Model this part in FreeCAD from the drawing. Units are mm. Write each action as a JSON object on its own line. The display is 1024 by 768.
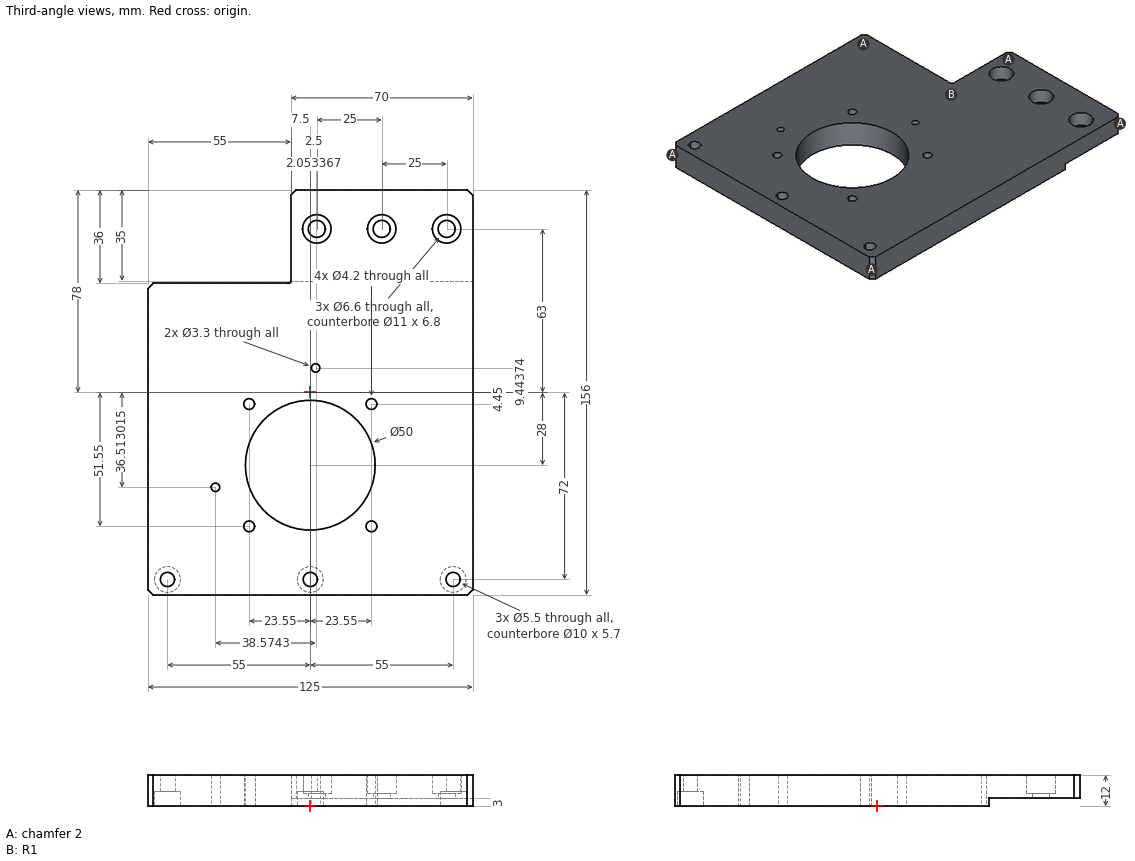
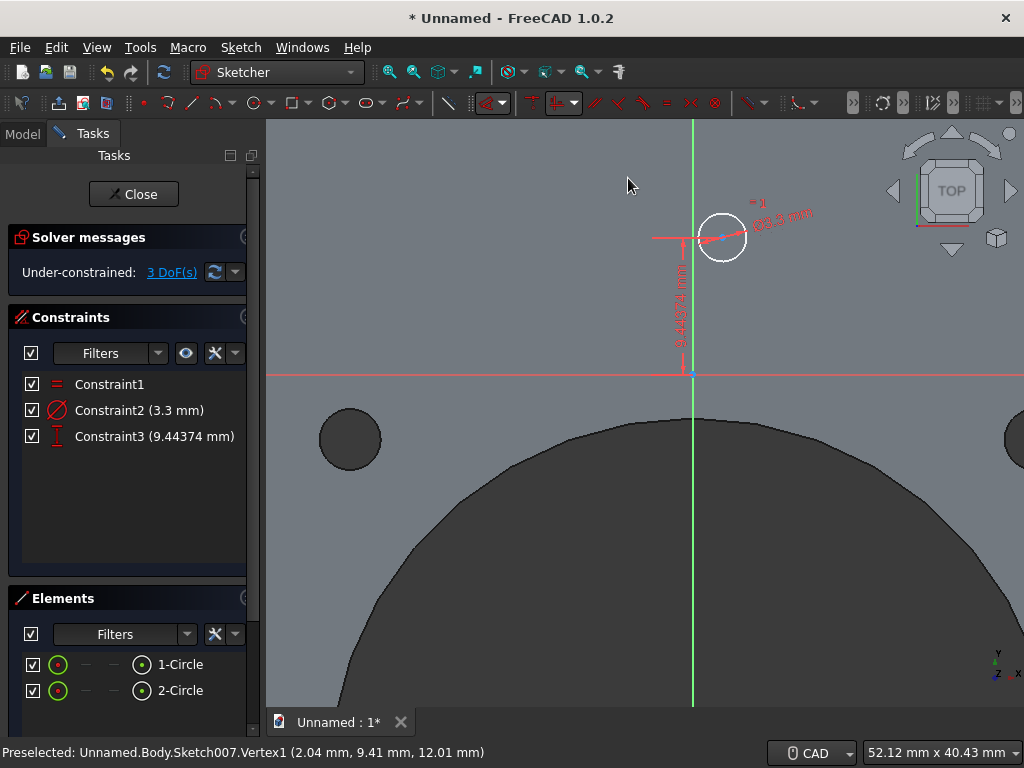
{"action": "scroll", "coordinate": [722, 238], "scroll_direction": "up", "scroll_amount": 2}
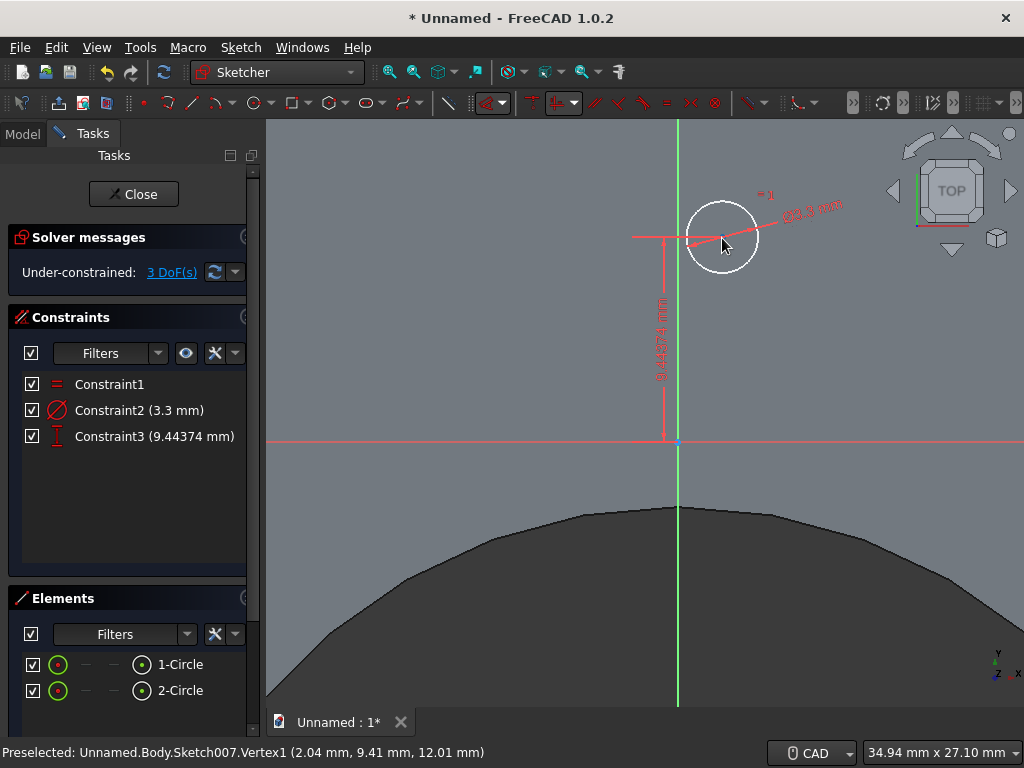
{"action": "left_click", "coordinate": [722, 237]}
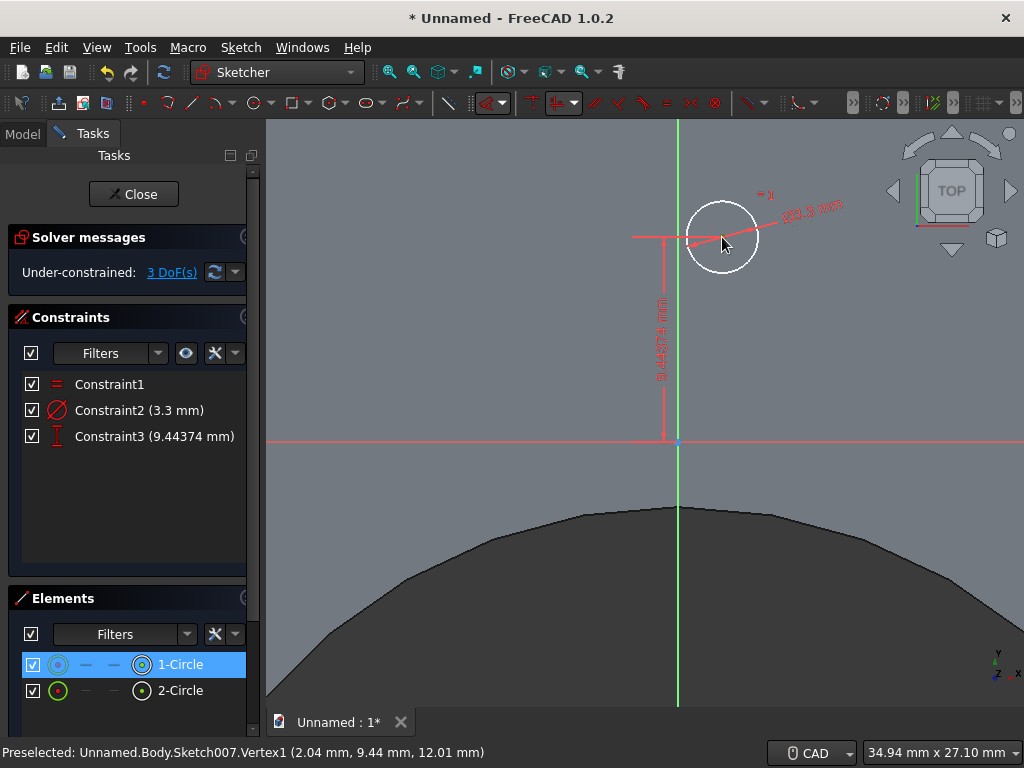
{"action": "left_click", "coordinate": [504, 104]}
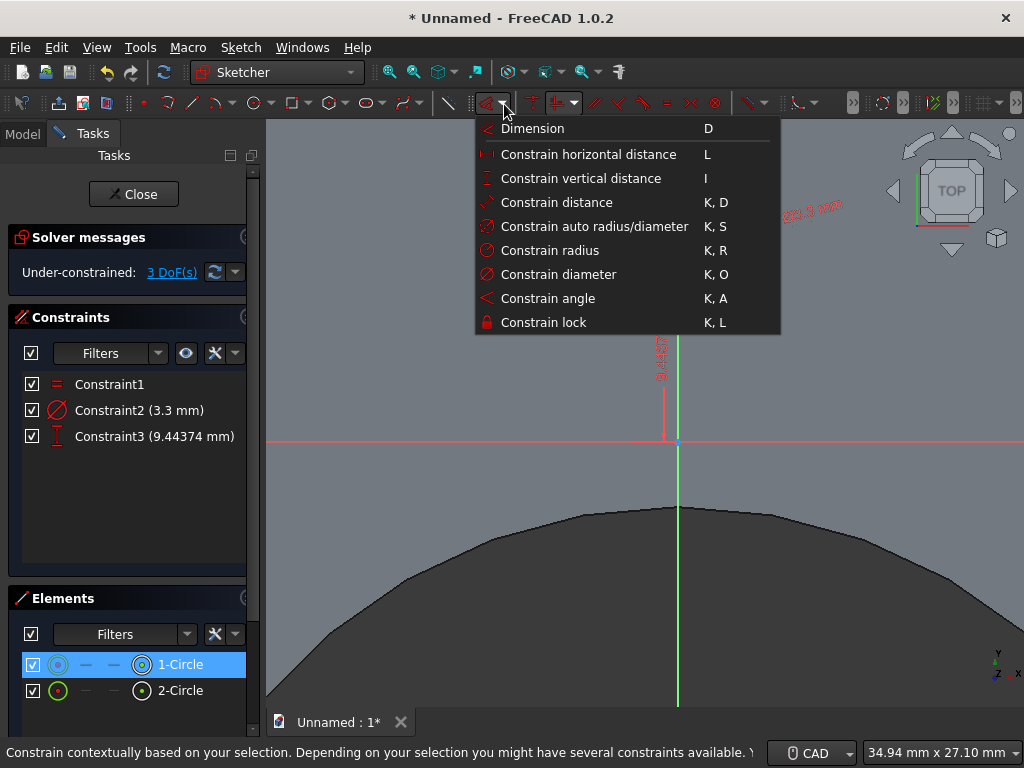
{"action": "left_click", "coordinate": [628, 154]}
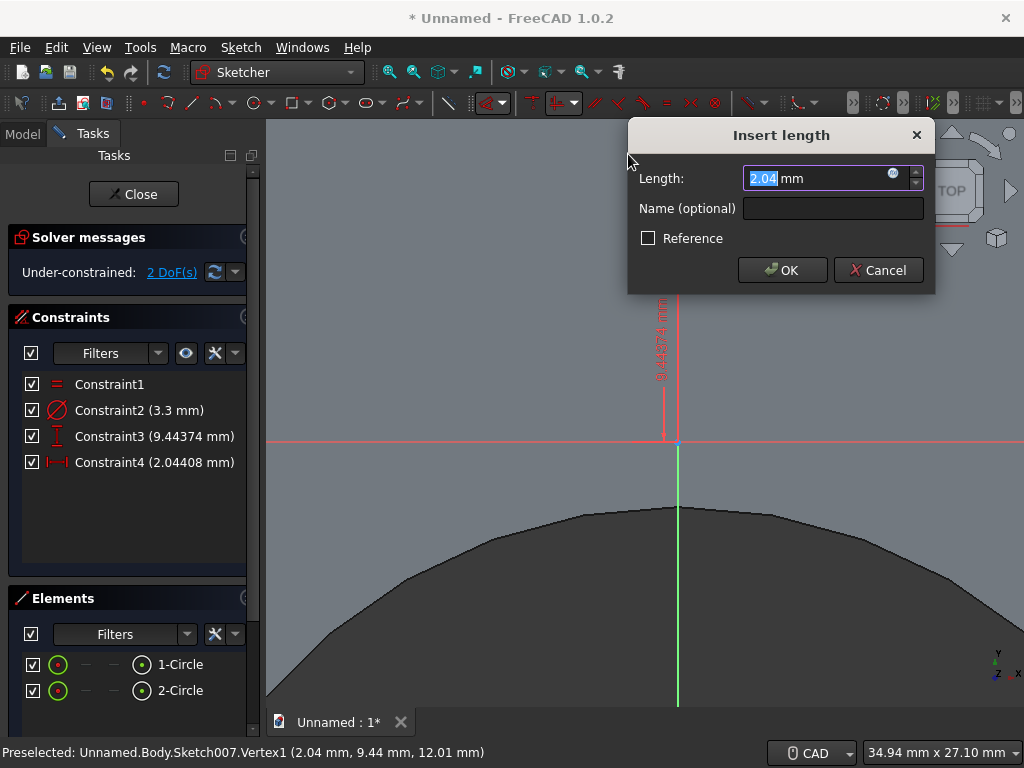
{"action": "type", "text": "2.053367"}
{"action": "key", "text": "Return"}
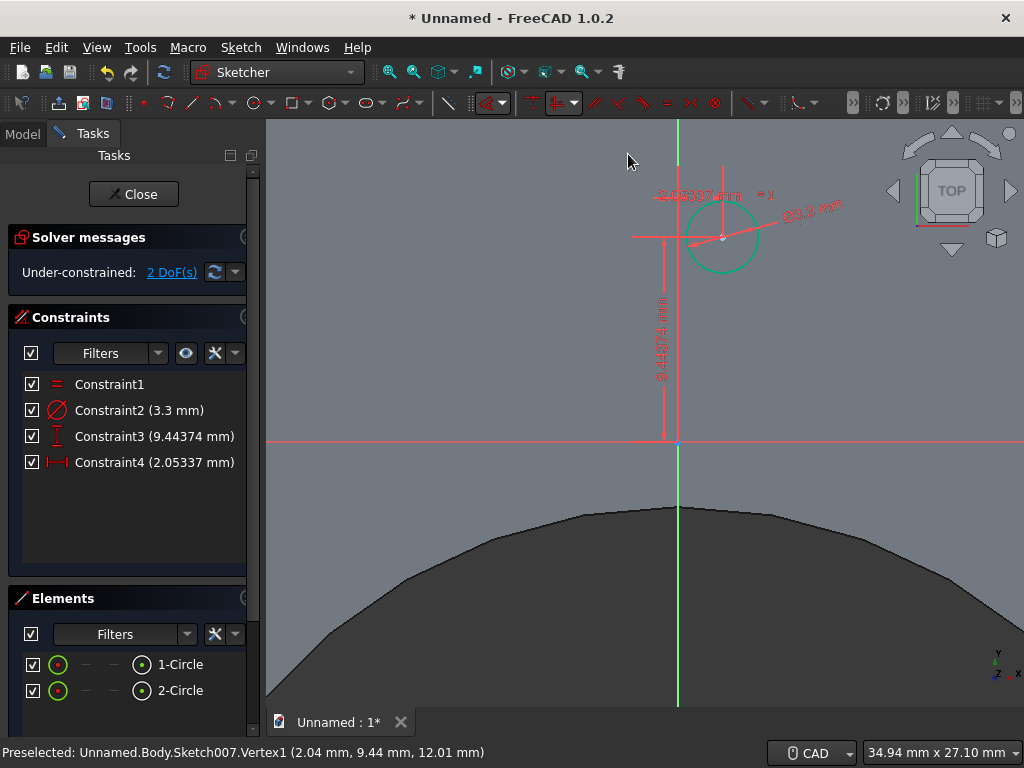
{"action": "left_click", "coordinate": [723, 237]}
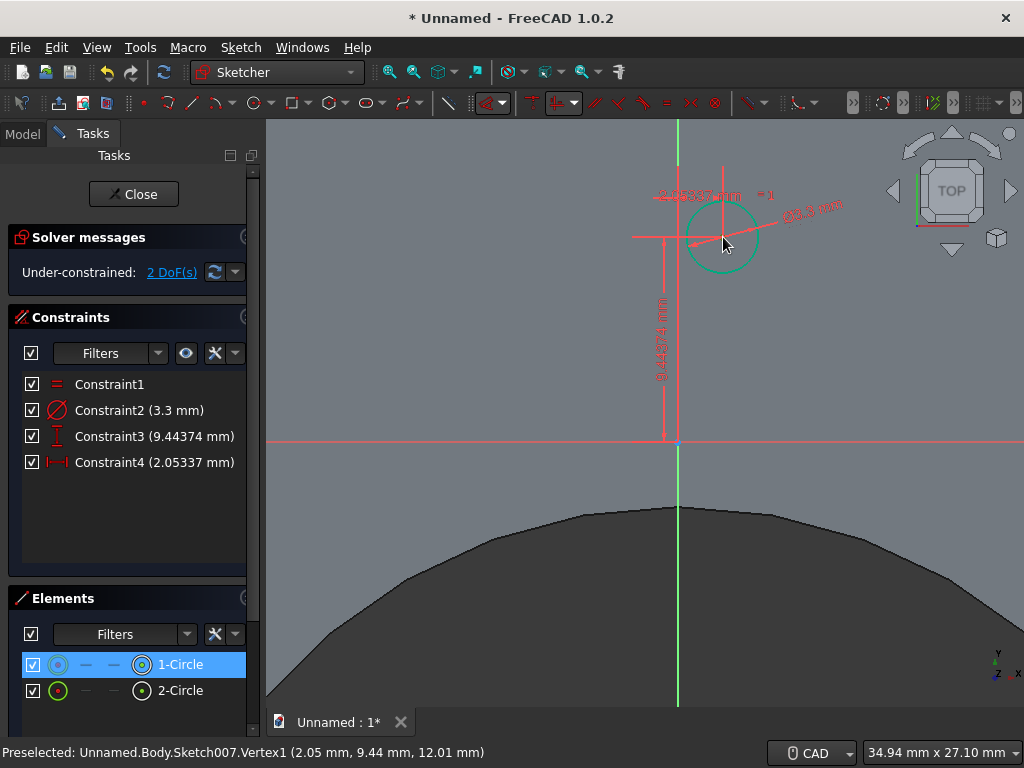
{"action": "scroll", "coordinate": [735, 225], "scroll_direction": "down", "scroll_amount": 5}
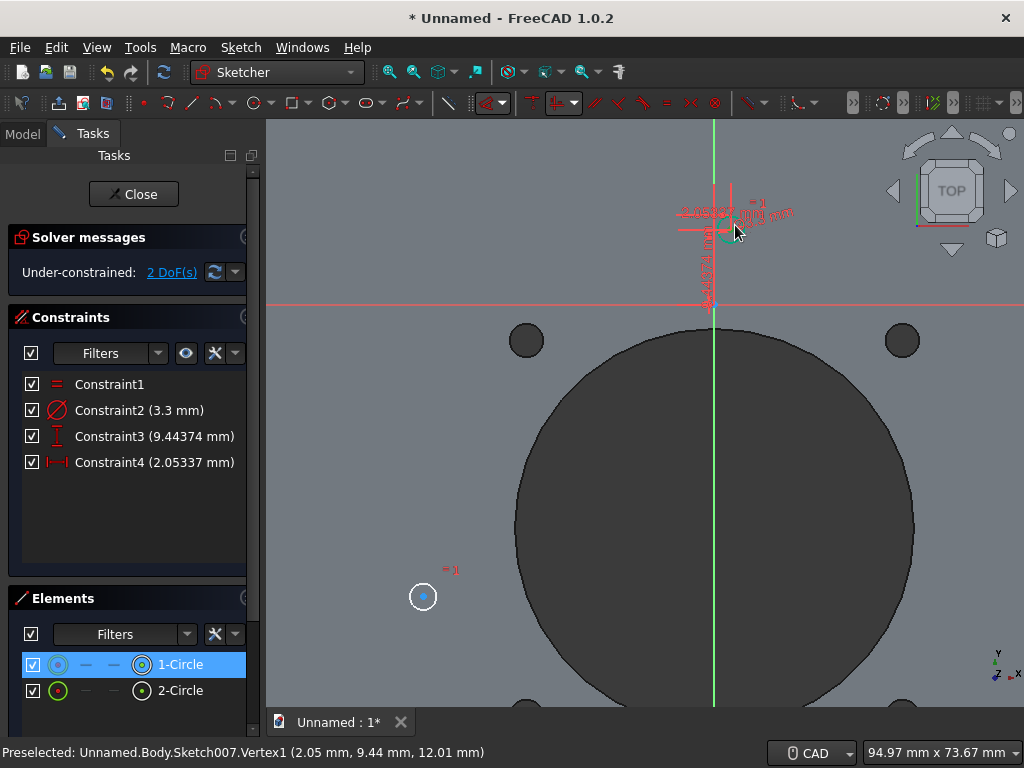
{"action": "left_click", "coordinate": [423, 597]}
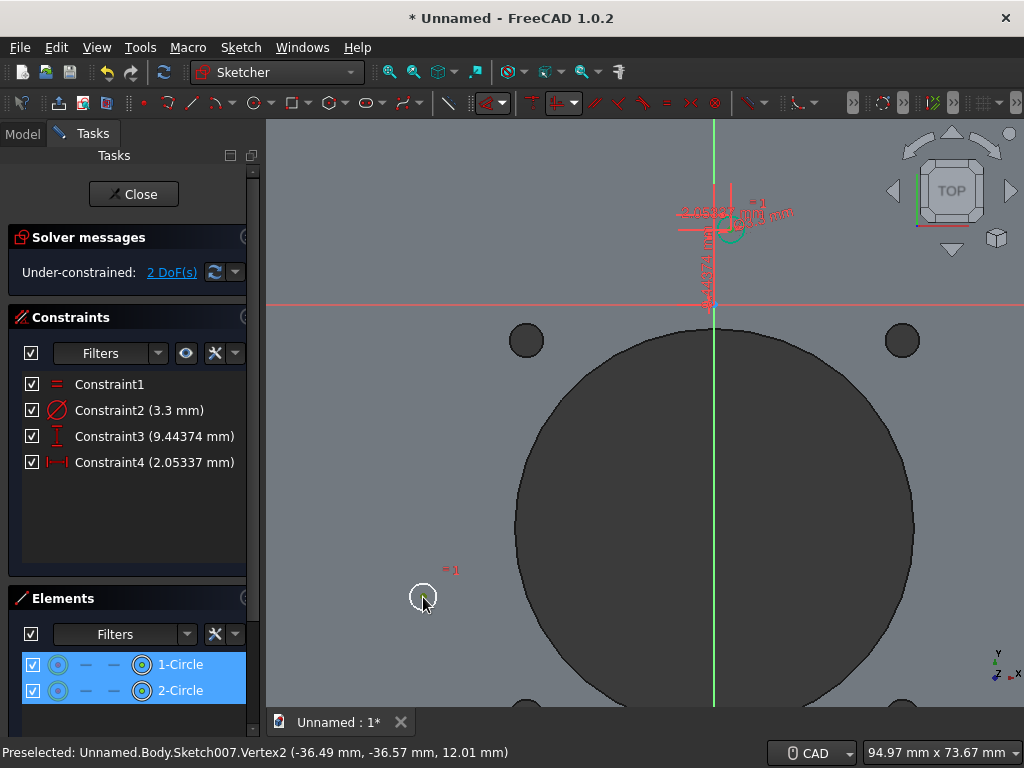
{"action": "left_click", "coordinate": [504, 104]}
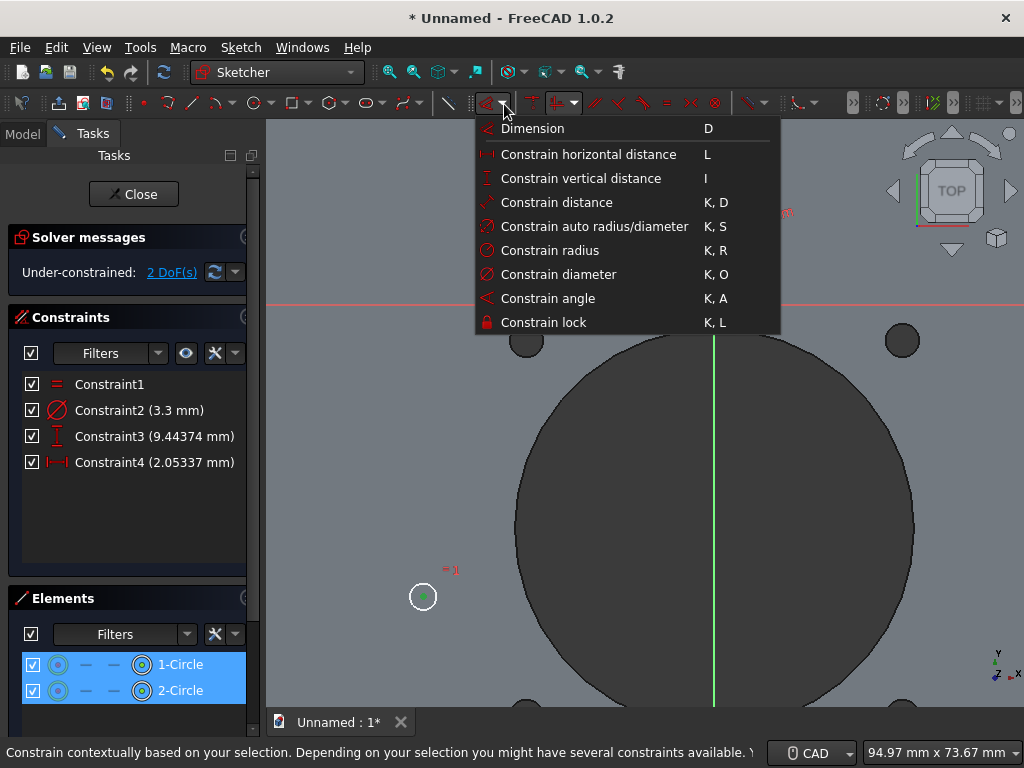
{"action": "left_click", "coordinate": [628, 154]}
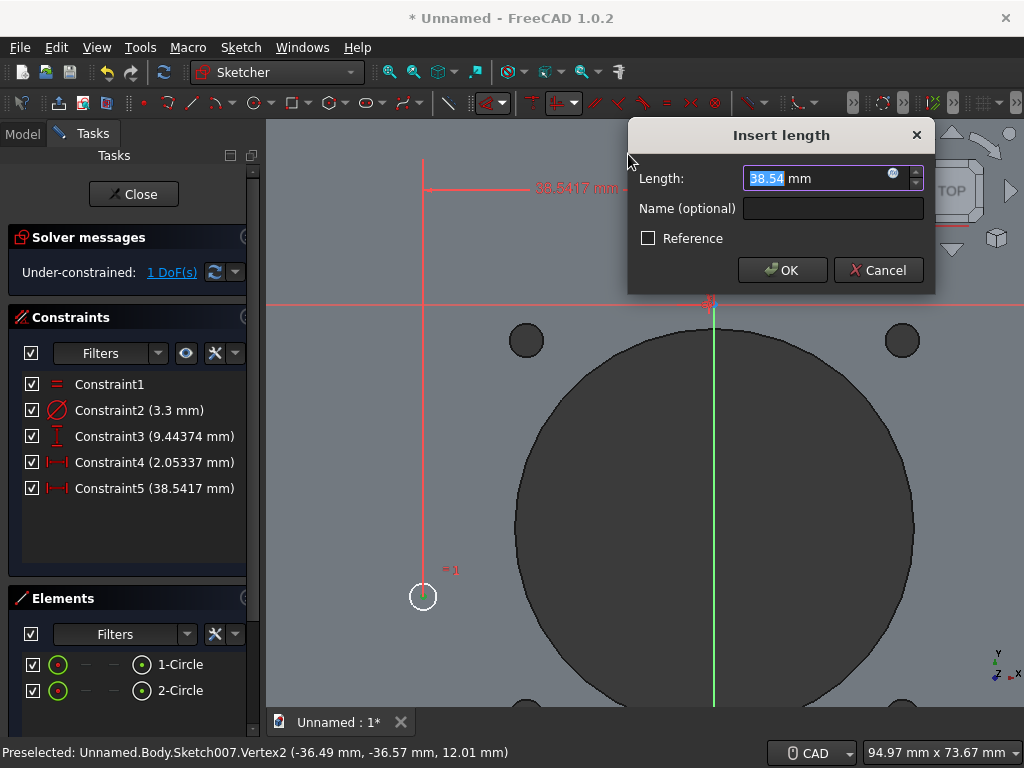
{"action": "type", "text": "38.5743"}
{"action": "key", "text": "Return"}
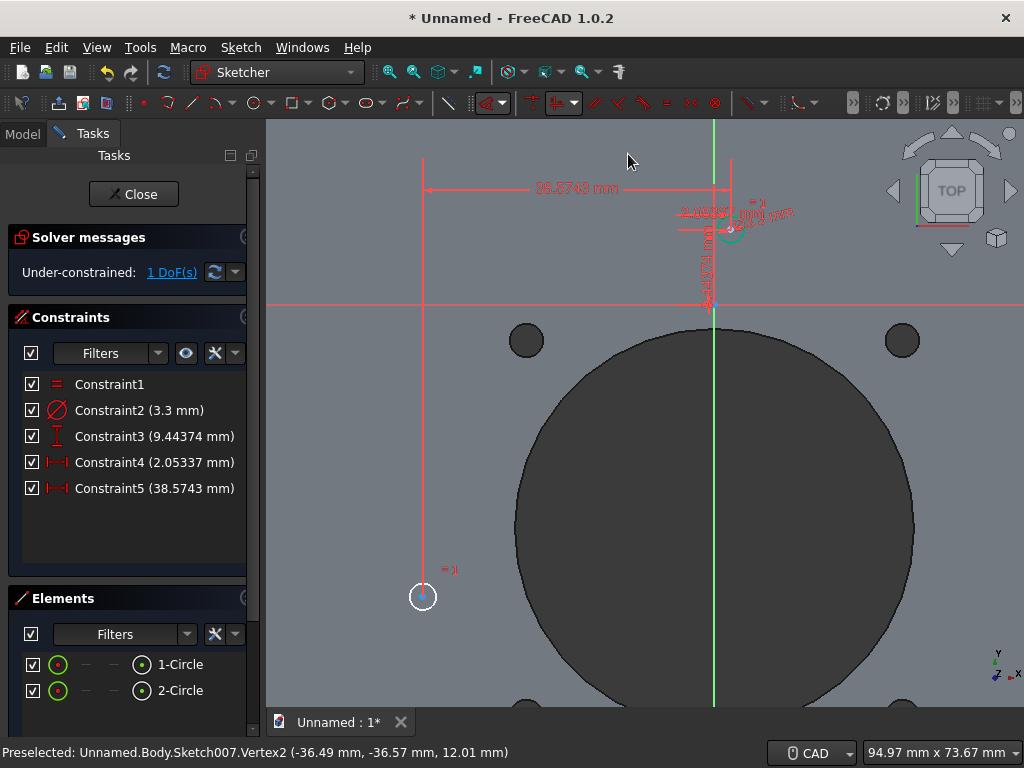
{"action": "left_click", "coordinate": [423, 597]}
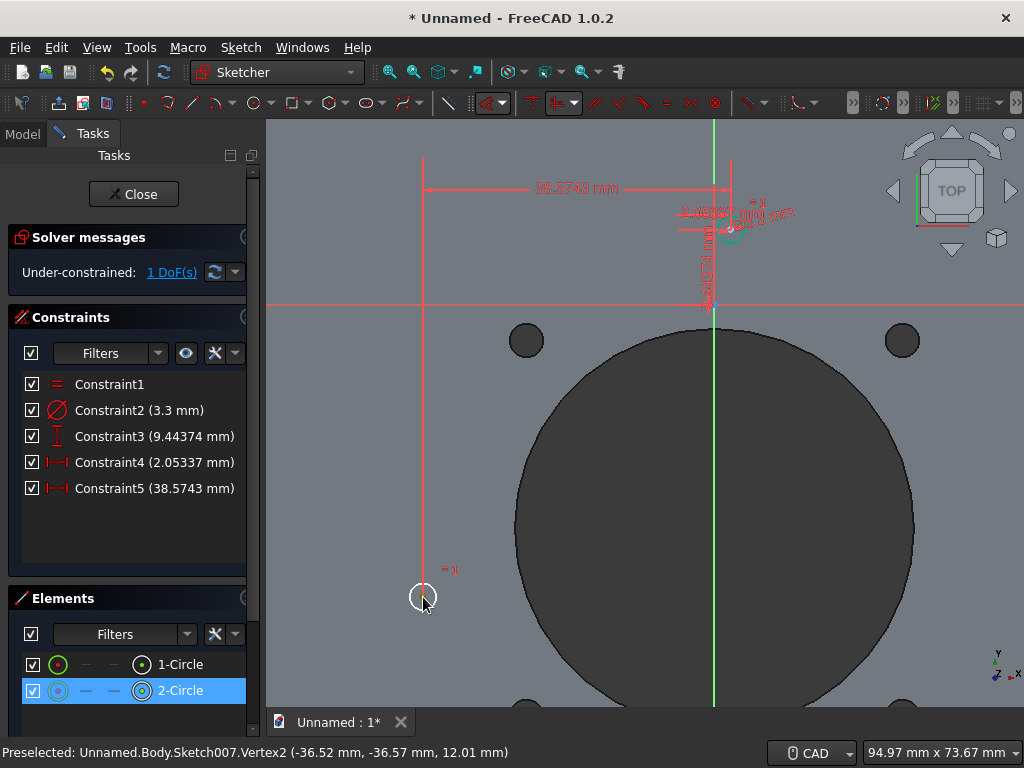
{"action": "key", "text": "i"}